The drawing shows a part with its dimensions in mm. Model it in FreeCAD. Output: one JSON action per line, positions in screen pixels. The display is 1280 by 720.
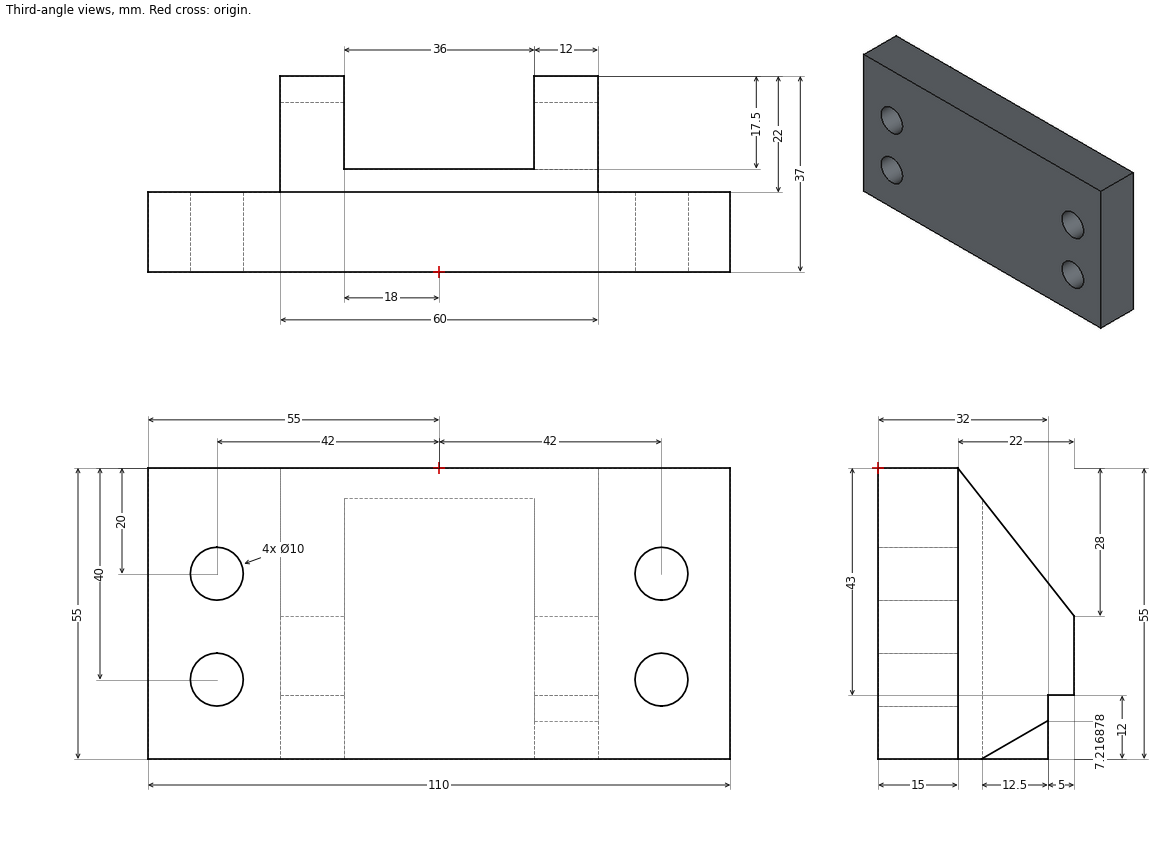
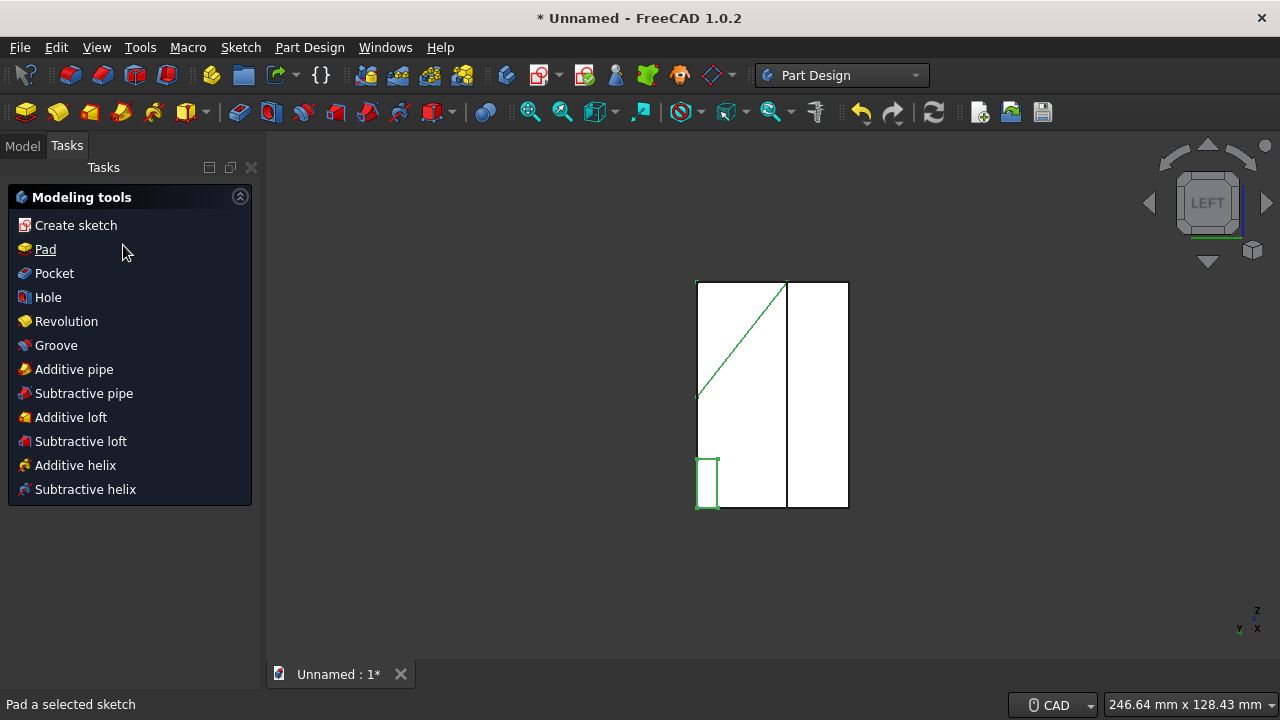
{"action": "left_click", "coordinate": [240, 112]}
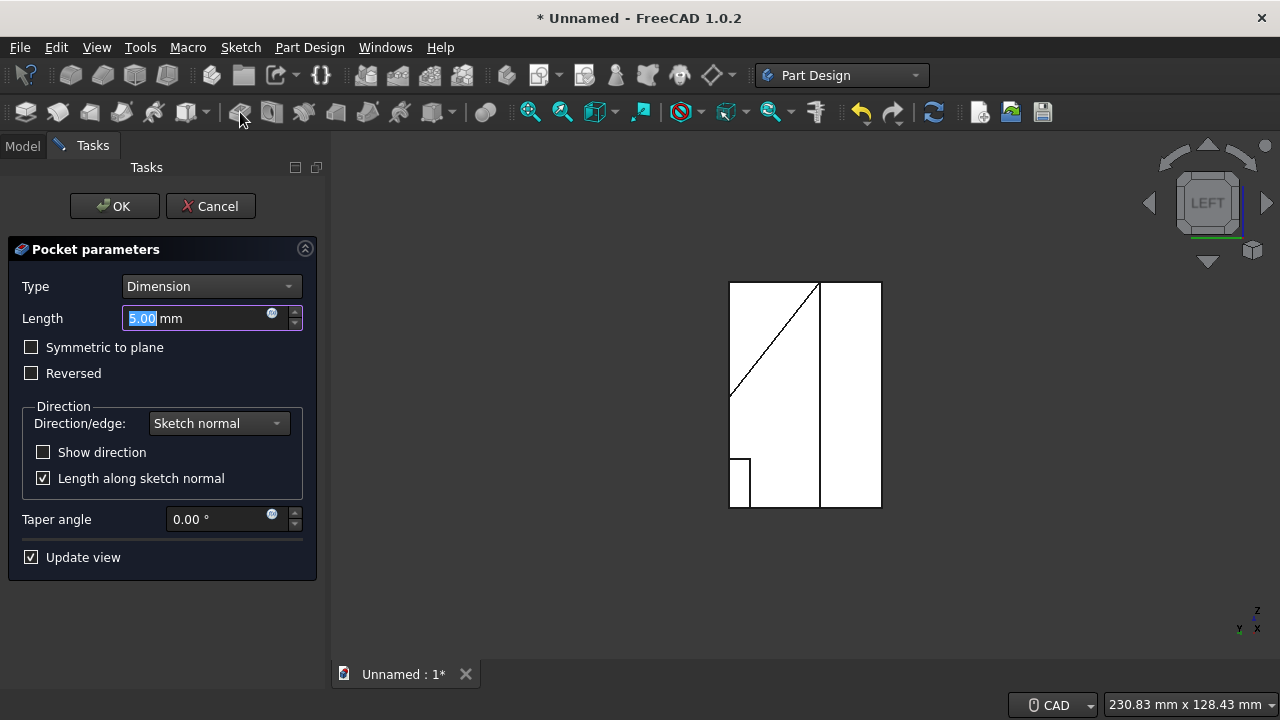
{"action": "left_click", "coordinate": [212, 286]}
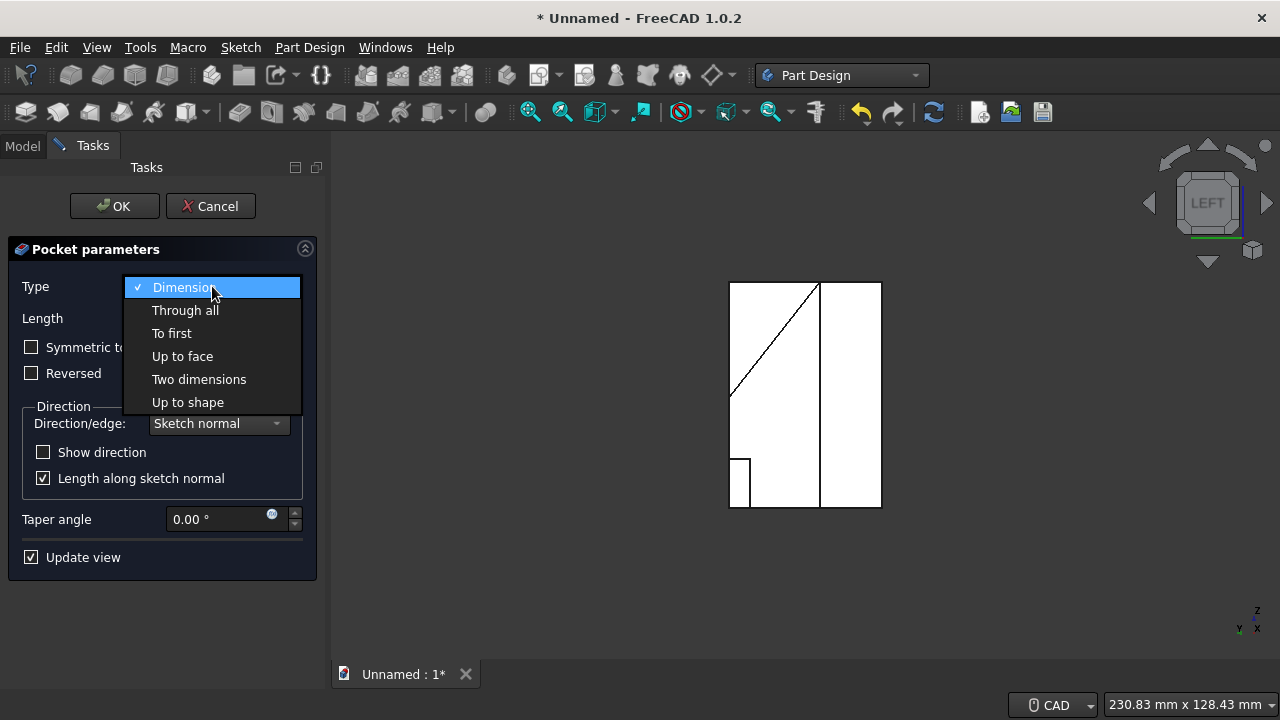
{"action": "left_click", "coordinate": [212, 310]}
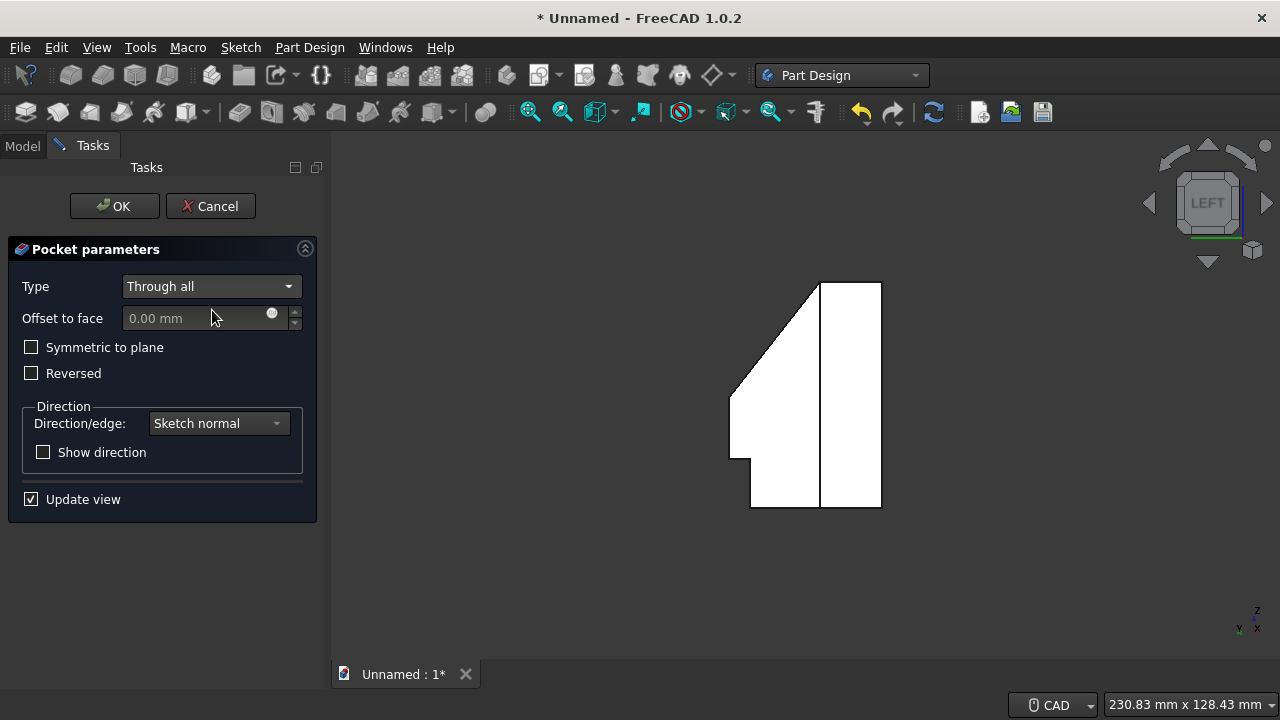
{"action": "left_click", "coordinate": [115, 206]}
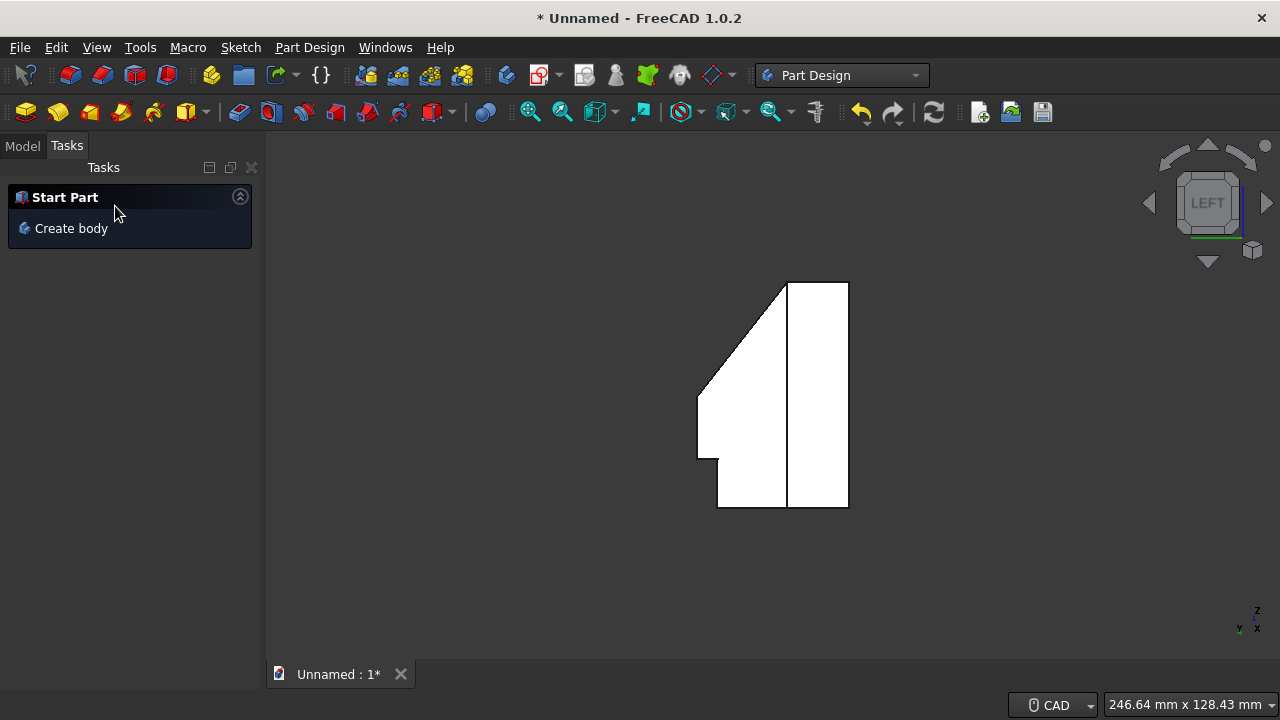
{"action": "left_click", "coordinate": [532, 112]}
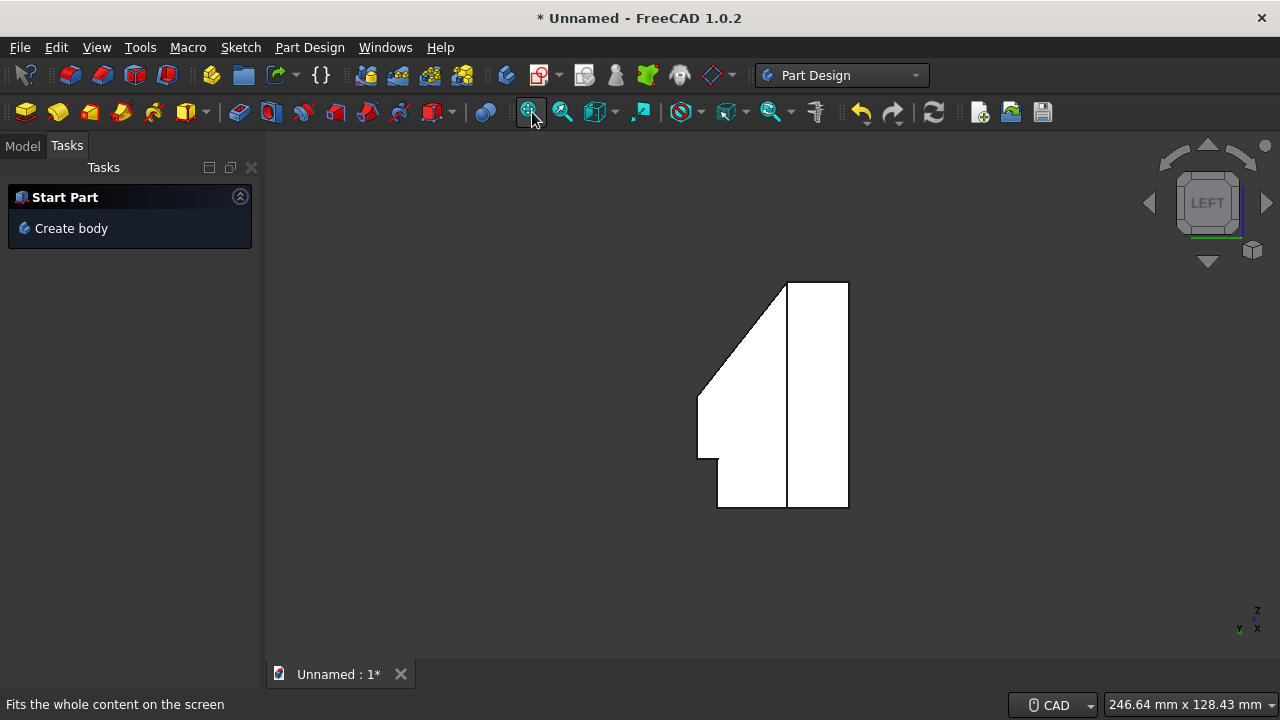
{"action": "left_click", "coordinate": [23, 145]}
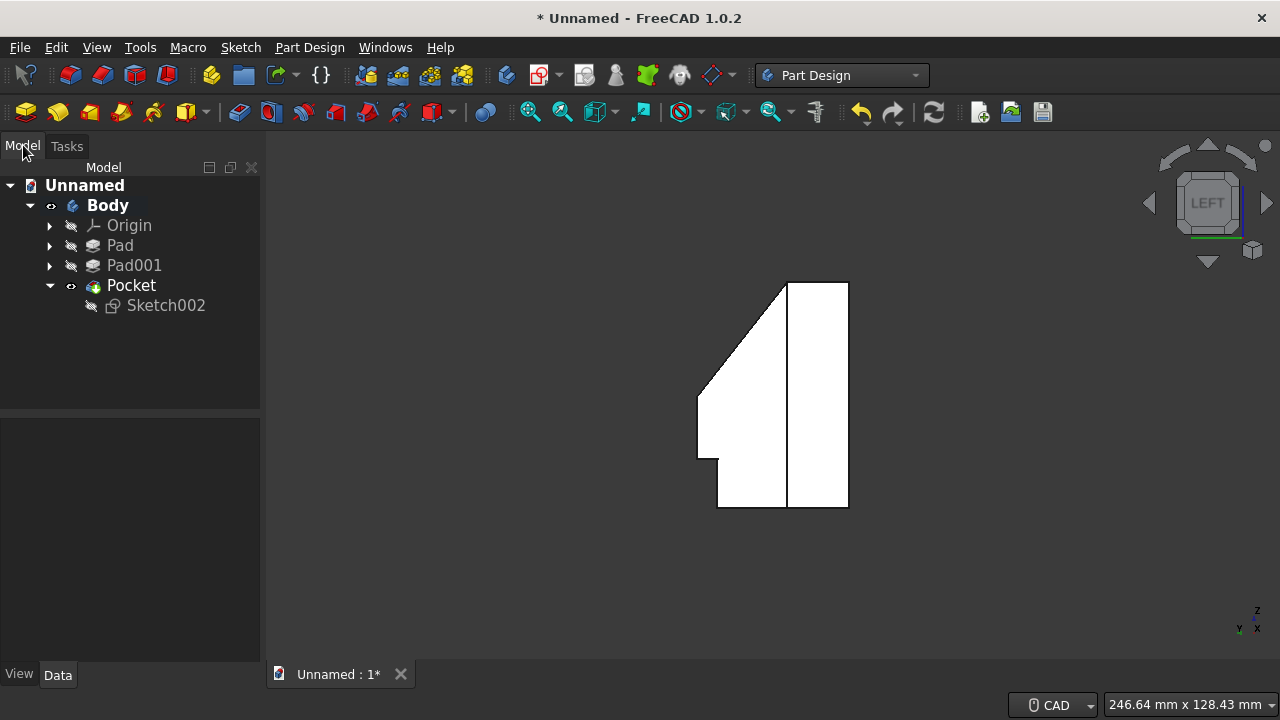
{"action": "left_click", "coordinate": [50, 226]}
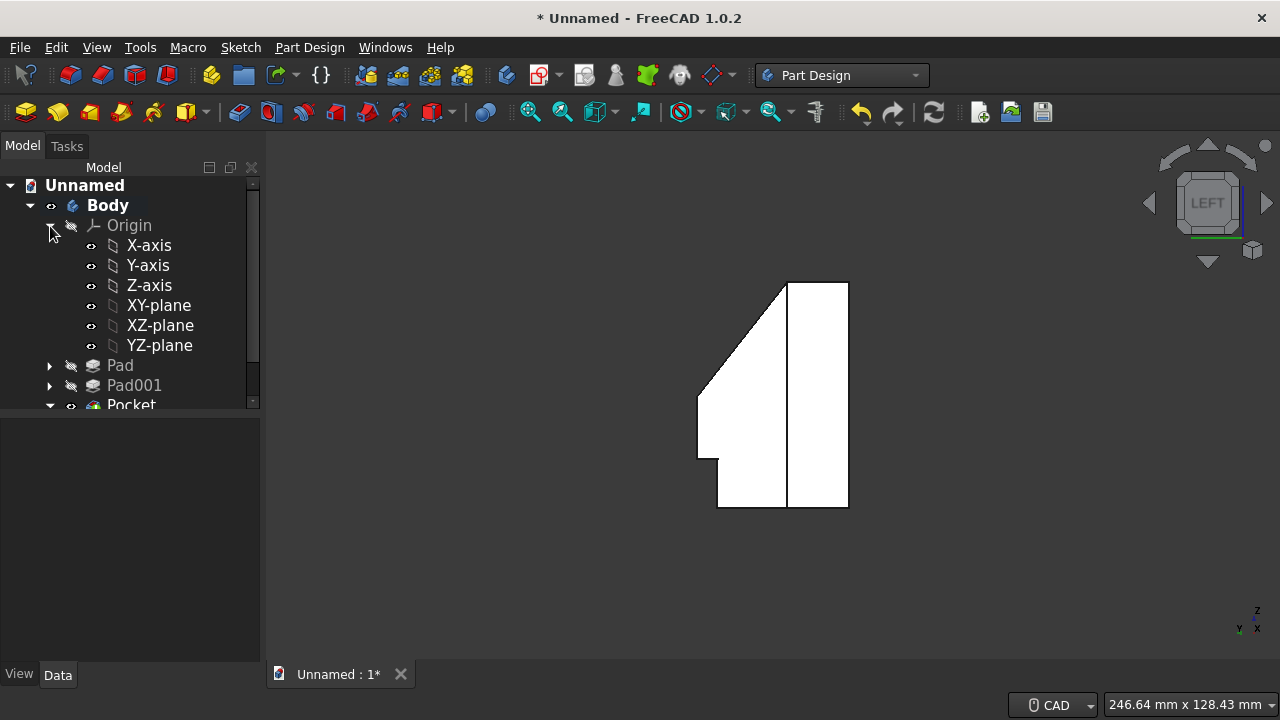
{"action": "left_click", "coordinate": [136, 346]}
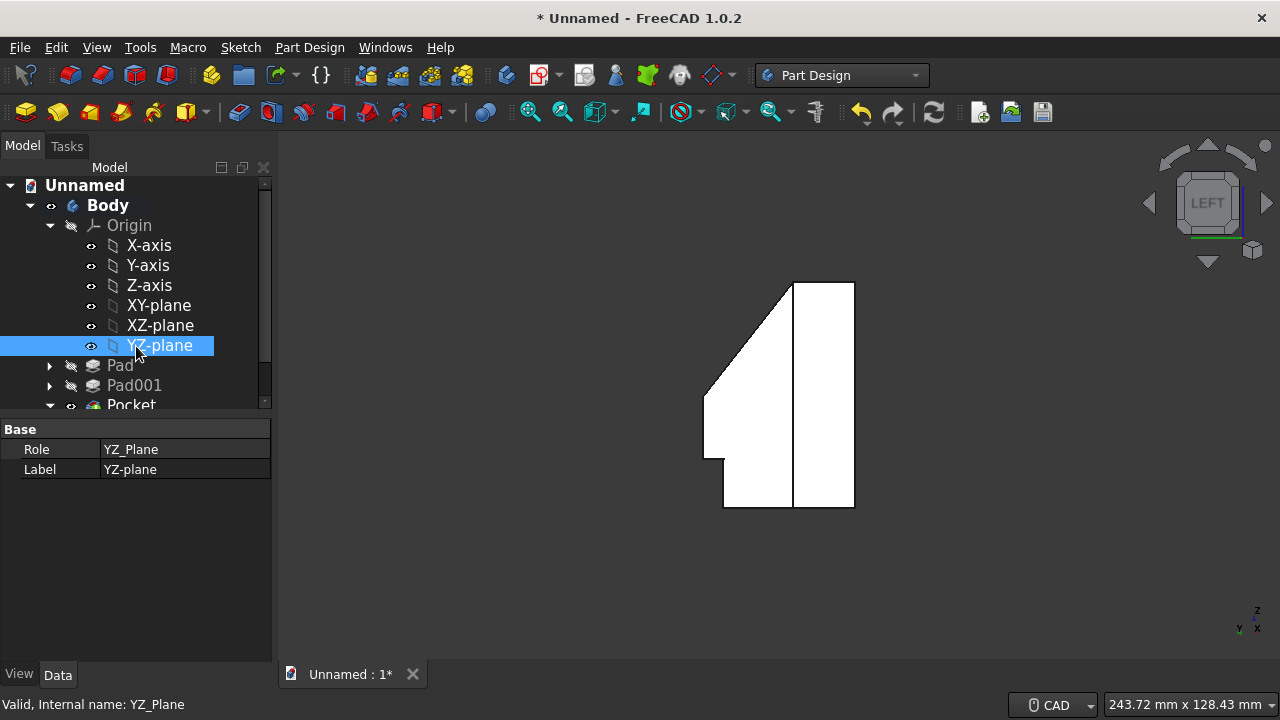
{"action": "left_click", "coordinate": [712, 76]}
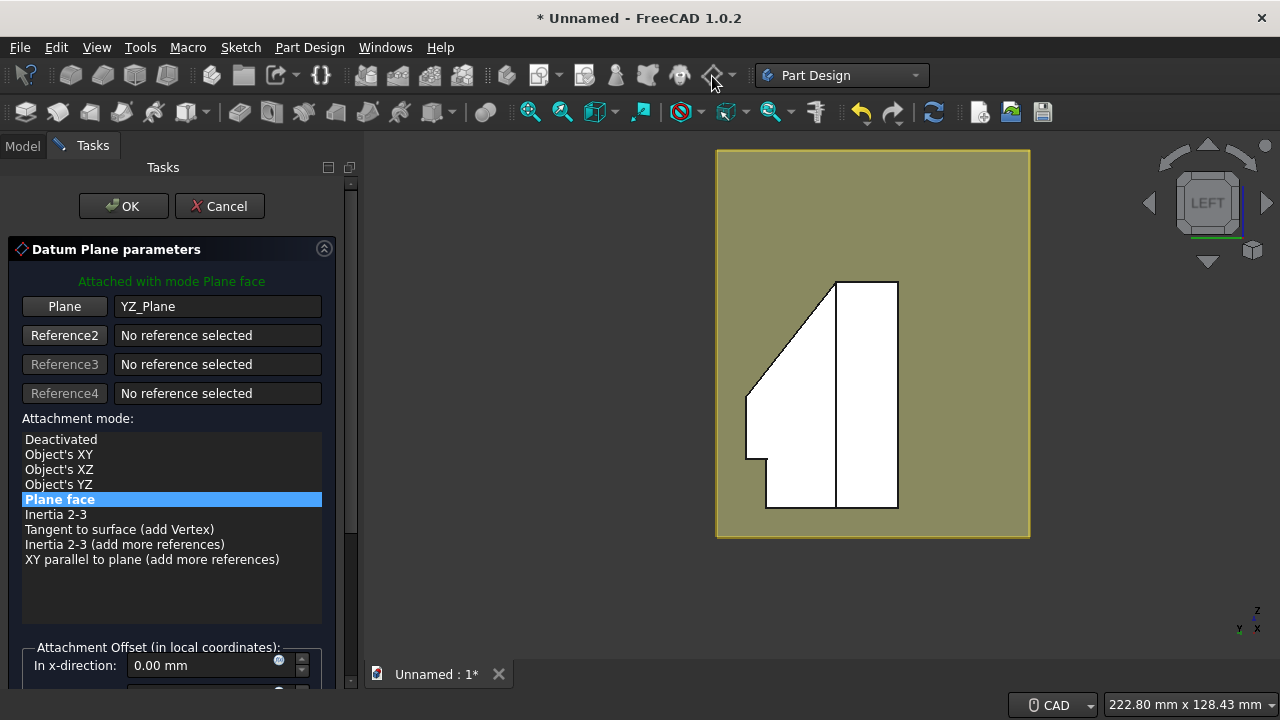
{"action": "scroll", "coordinate": [351, 432], "scroll_direction": "down", "scroll_amount": 2}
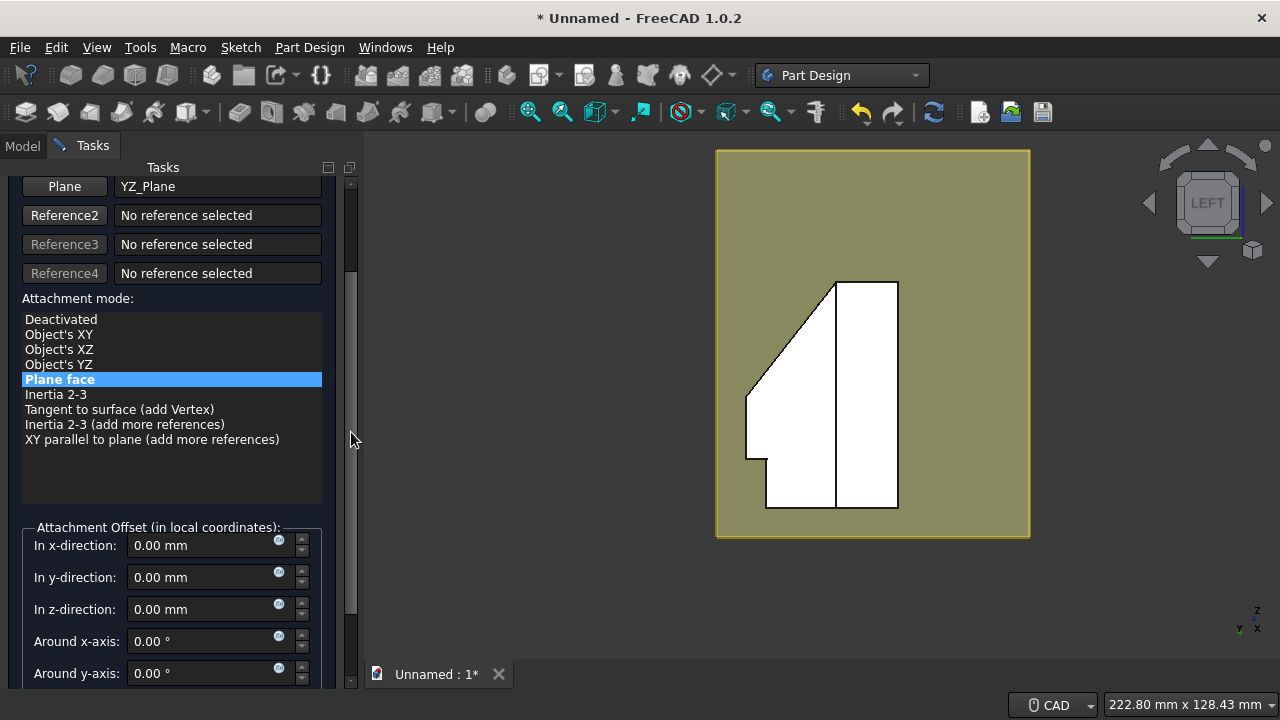
{"action": "triple_click", "coordinate": [210, 609]}